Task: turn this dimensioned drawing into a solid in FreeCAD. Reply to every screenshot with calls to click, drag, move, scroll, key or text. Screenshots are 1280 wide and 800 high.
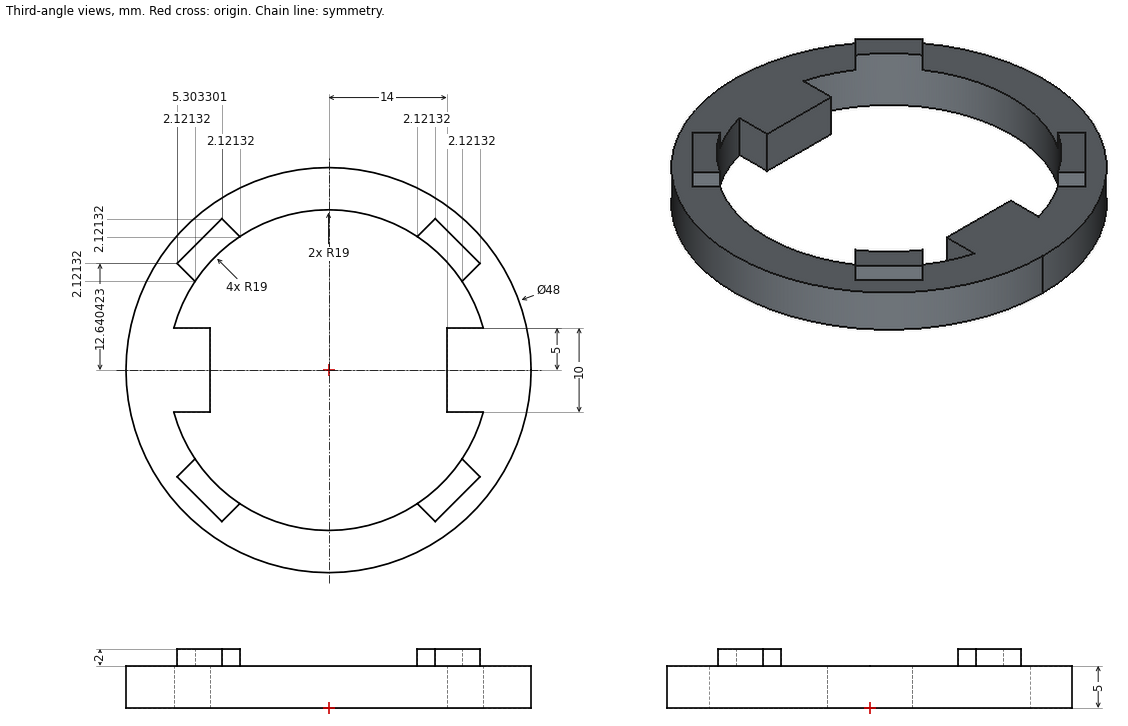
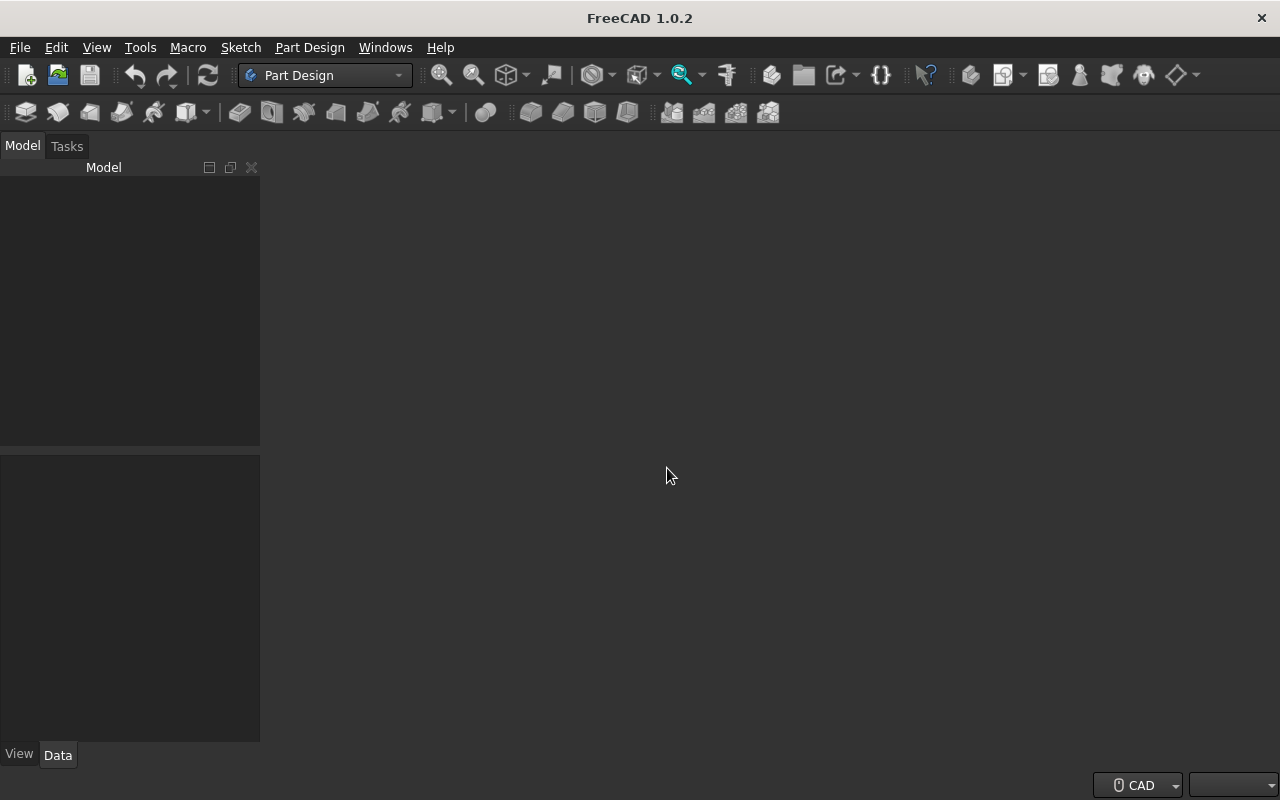
key(ctrl+n)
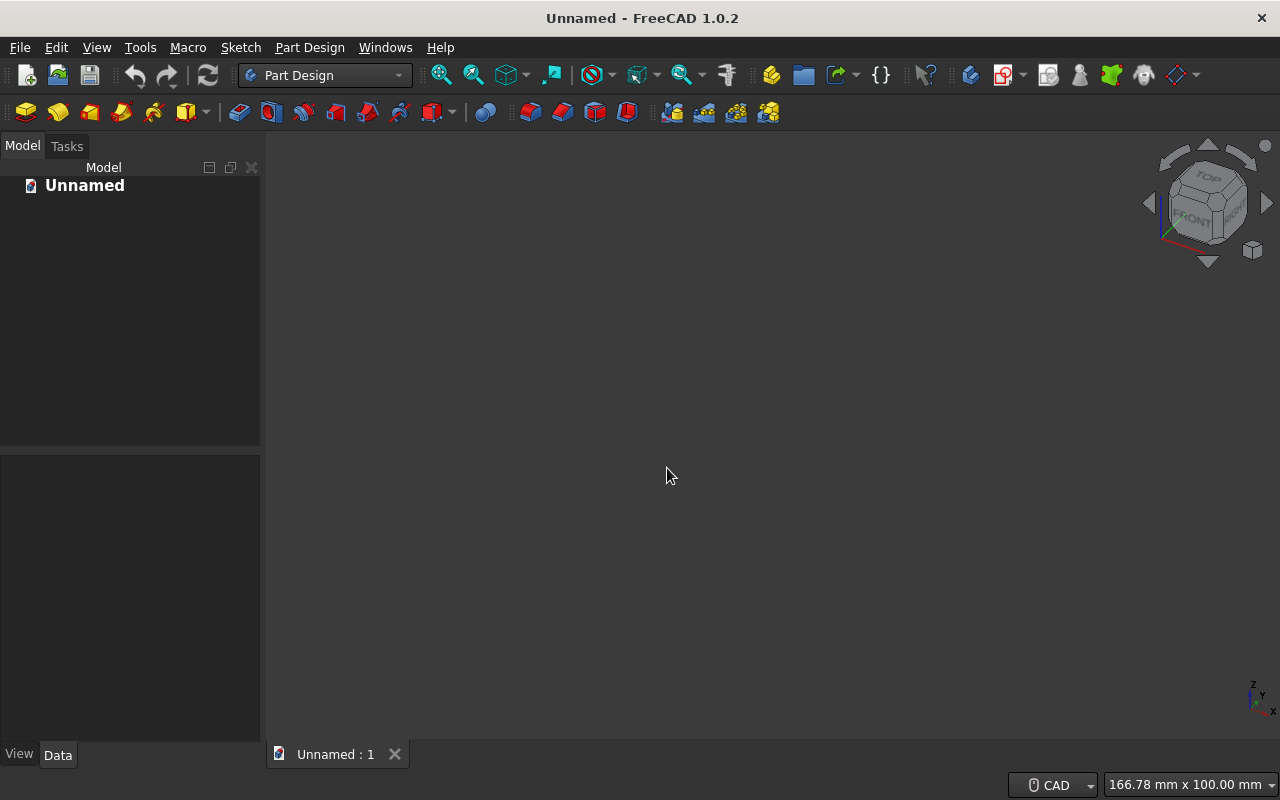
click(1004, 76)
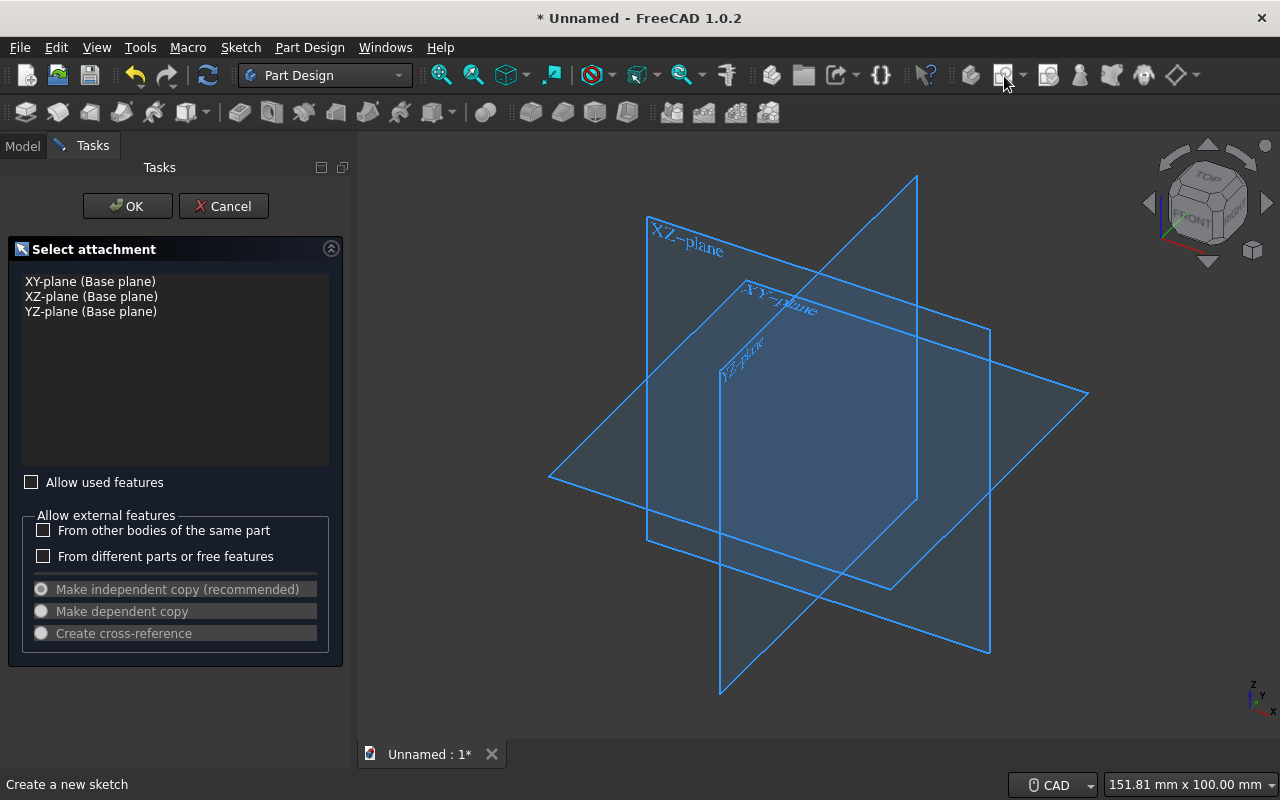
click(82, 282)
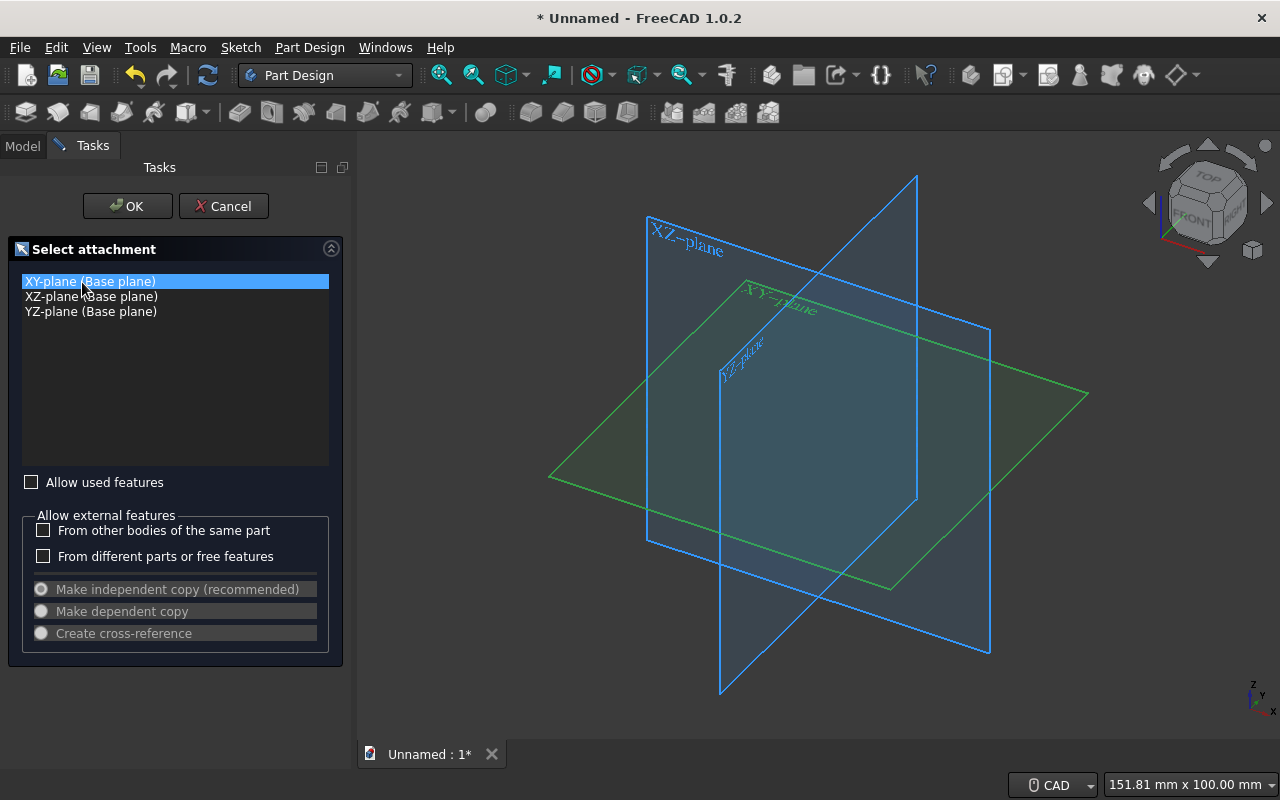
click(128, 206)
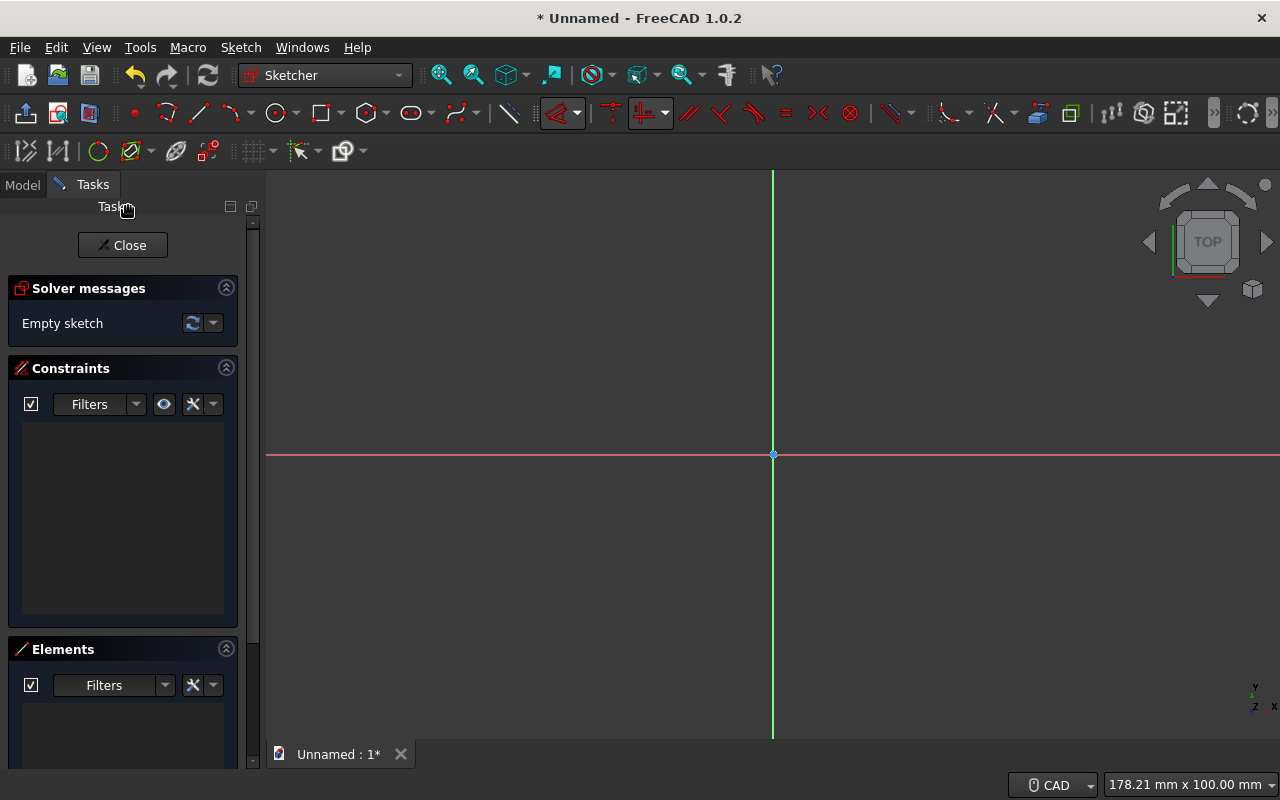
key(g)
key(m)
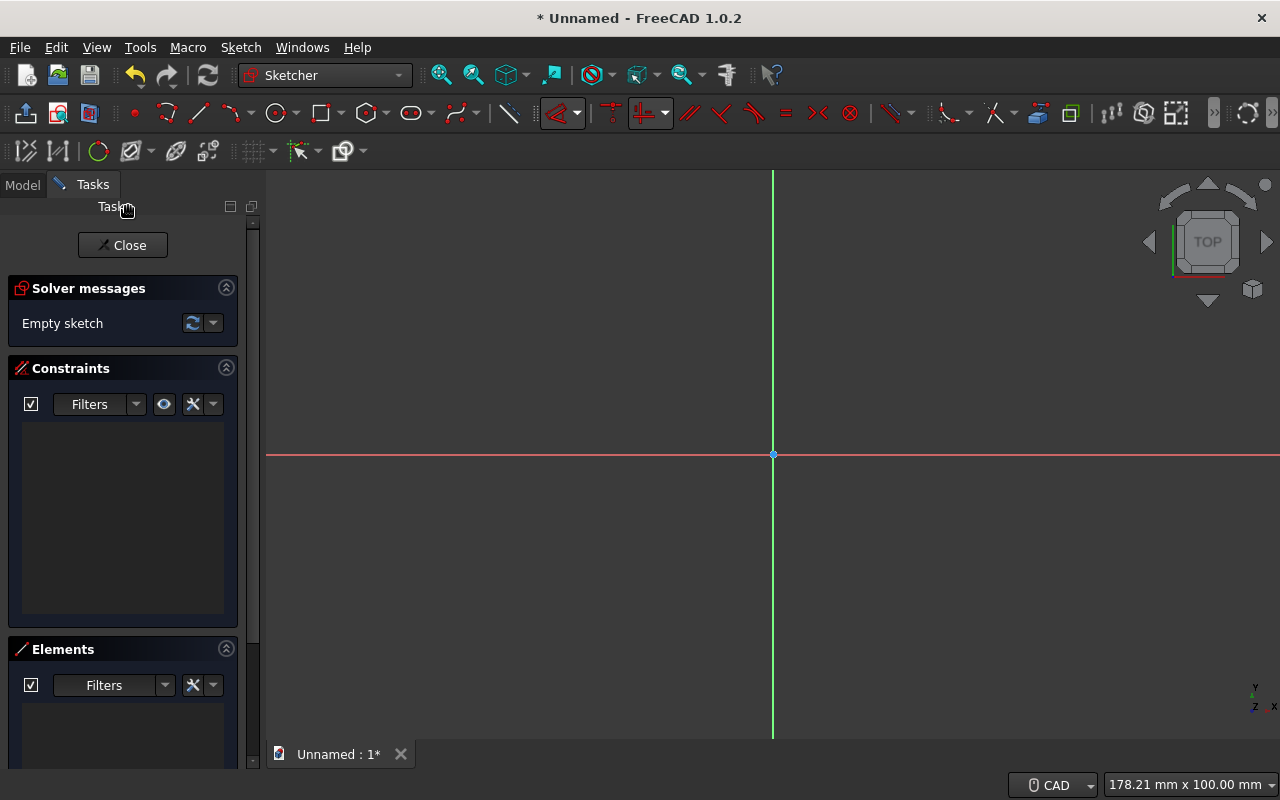
click(877, 426)
click(853, 426)
click(853, 483)
click(877, 483)
right_click(877, 483)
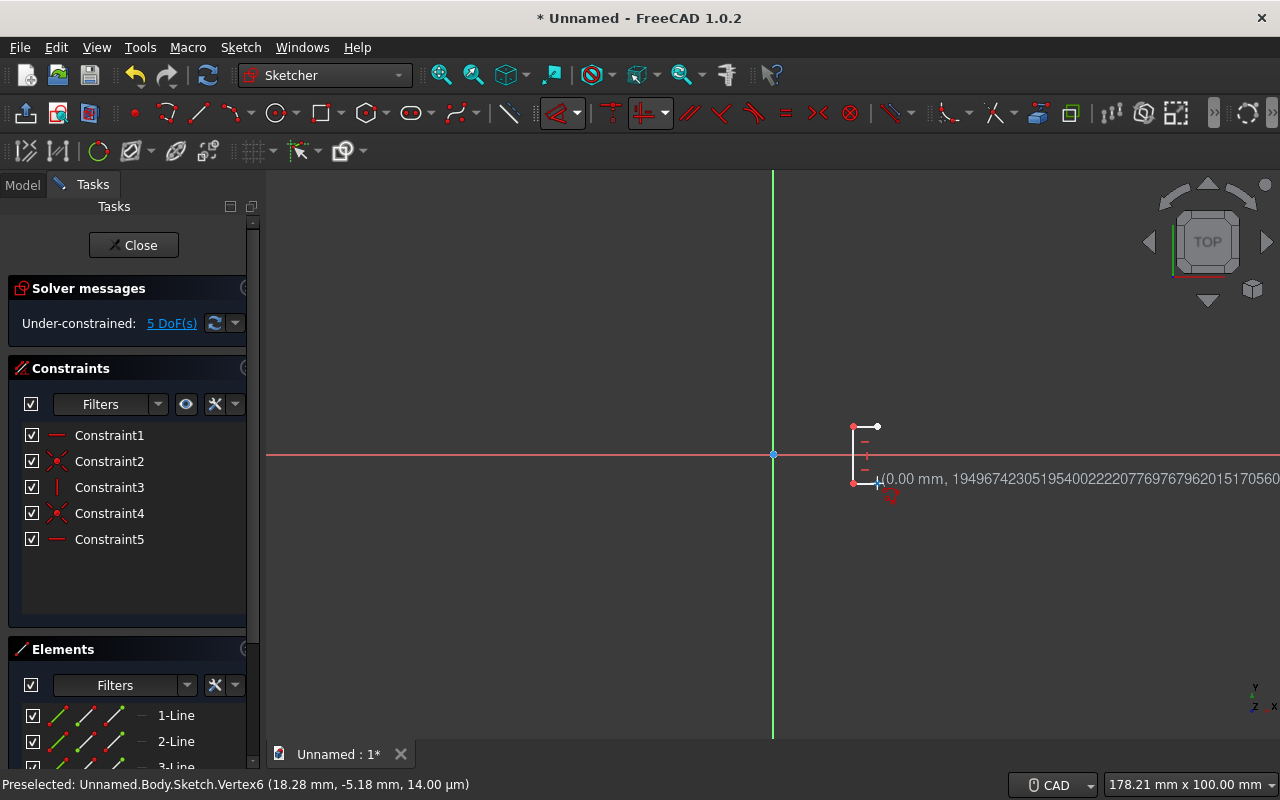
click(669, 483)
click(693, 483)
click(693, 426)
click(669, 426)
right_click(669, 426)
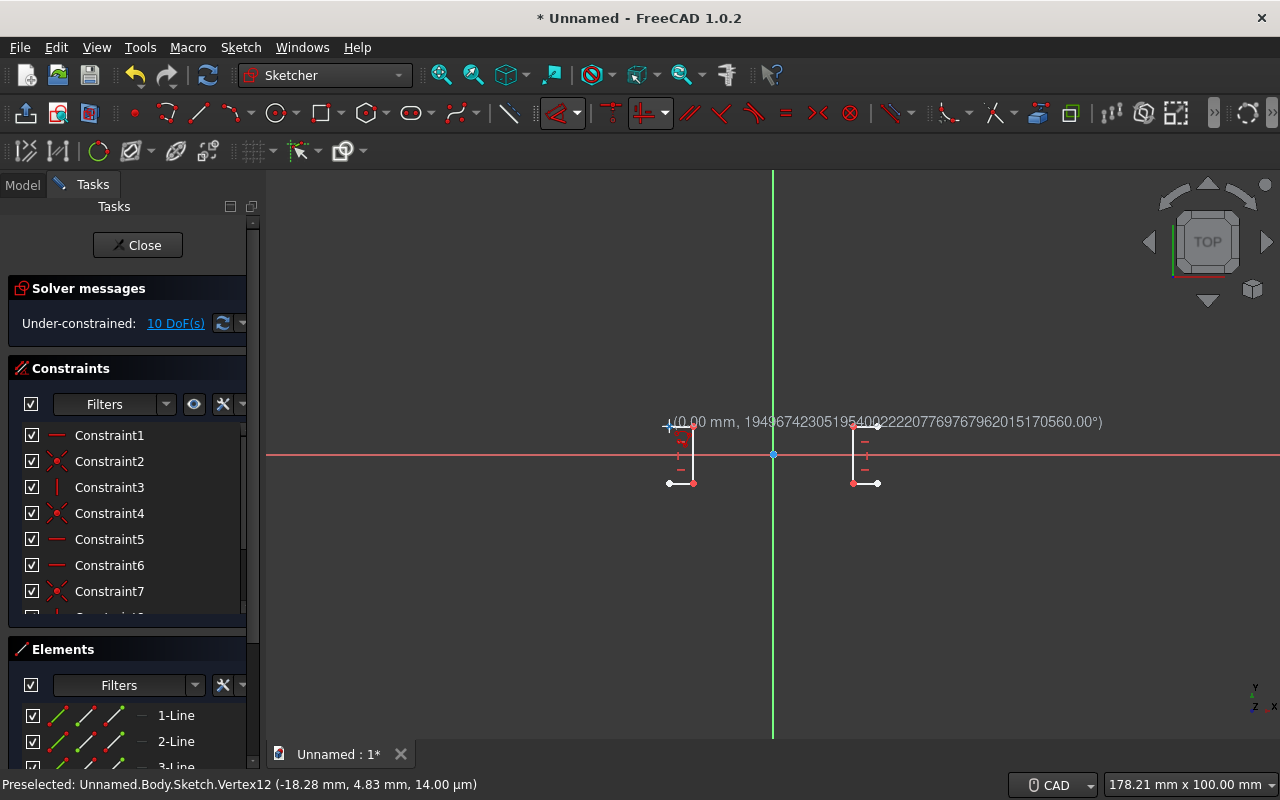
click(232, 114)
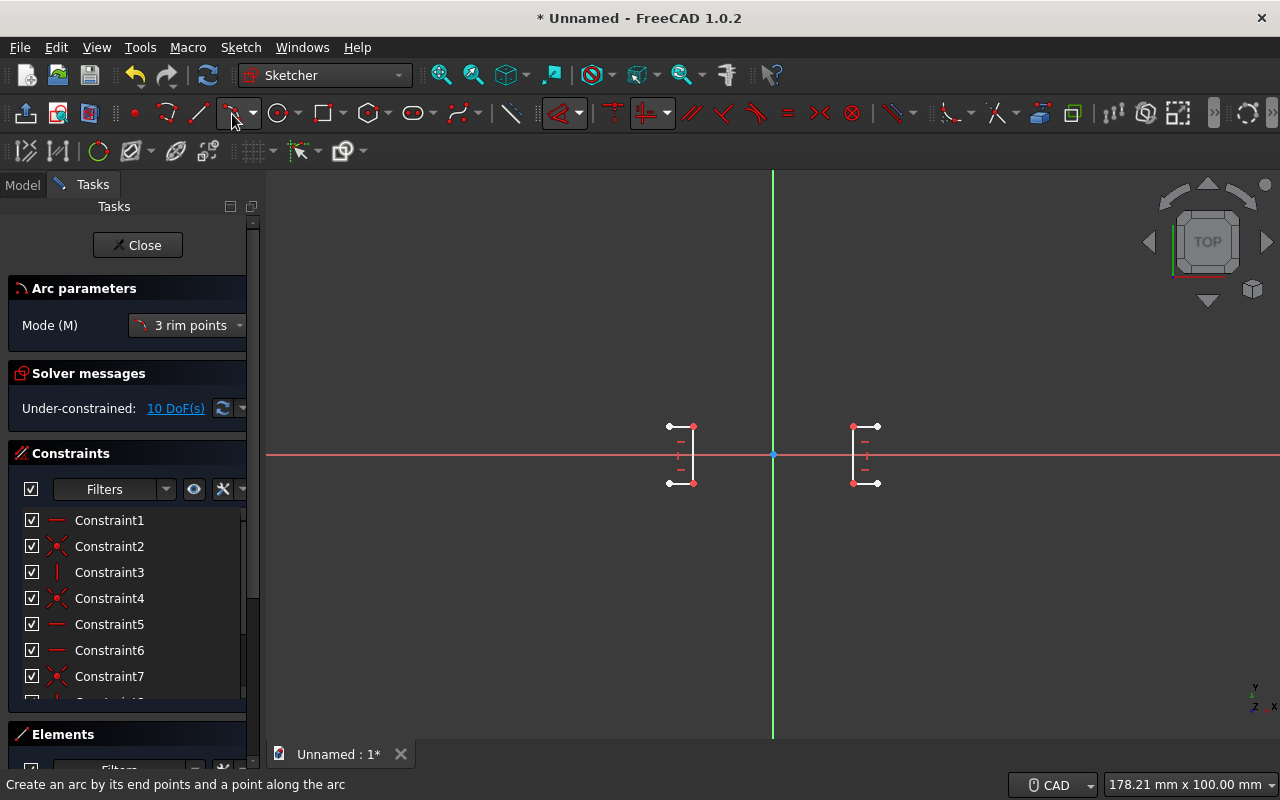
scroll(877, 483, up, 2)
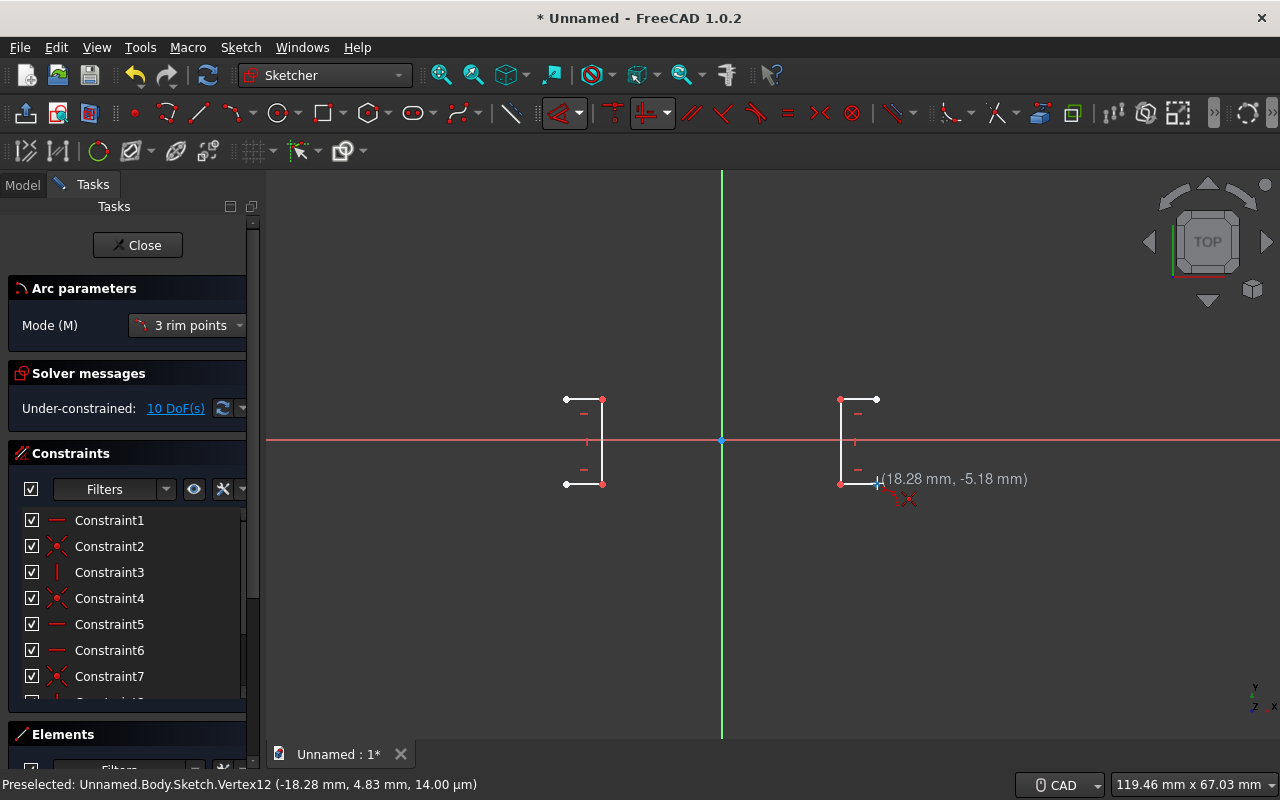
click(877, 484)
click(566, 484)
click(680, 596)